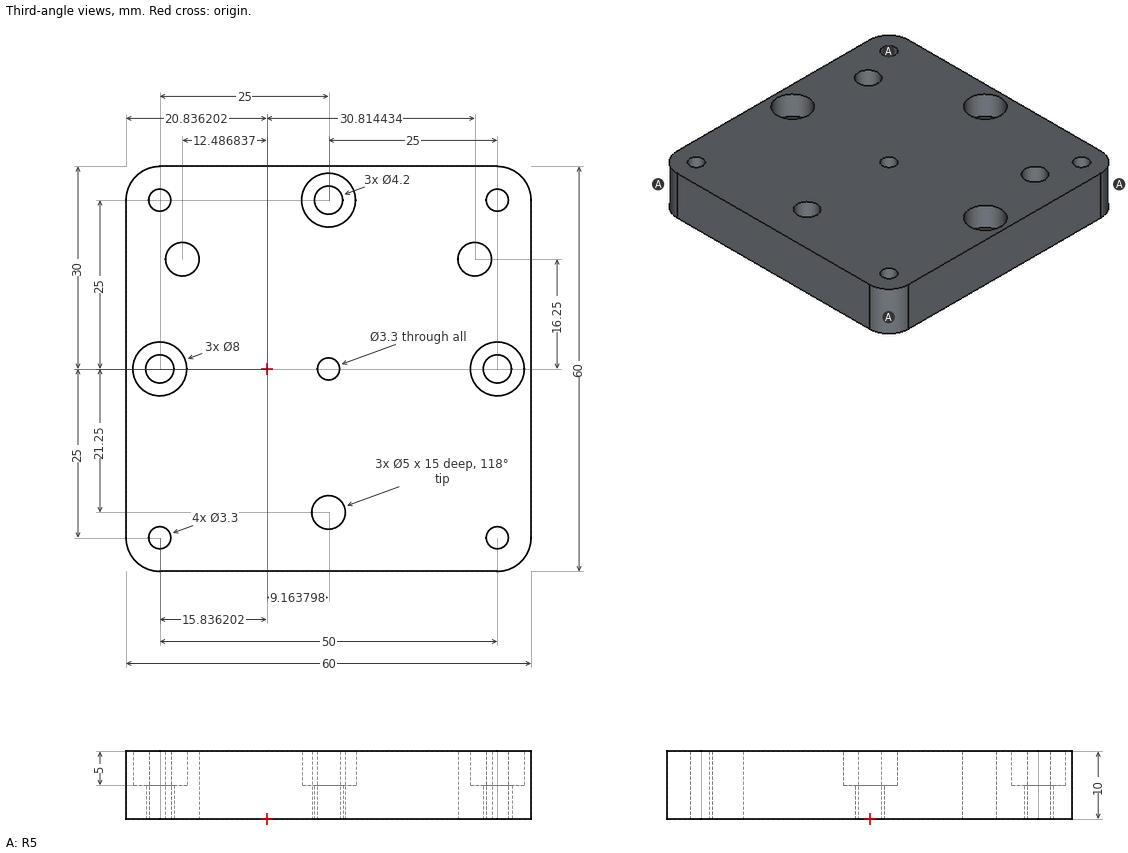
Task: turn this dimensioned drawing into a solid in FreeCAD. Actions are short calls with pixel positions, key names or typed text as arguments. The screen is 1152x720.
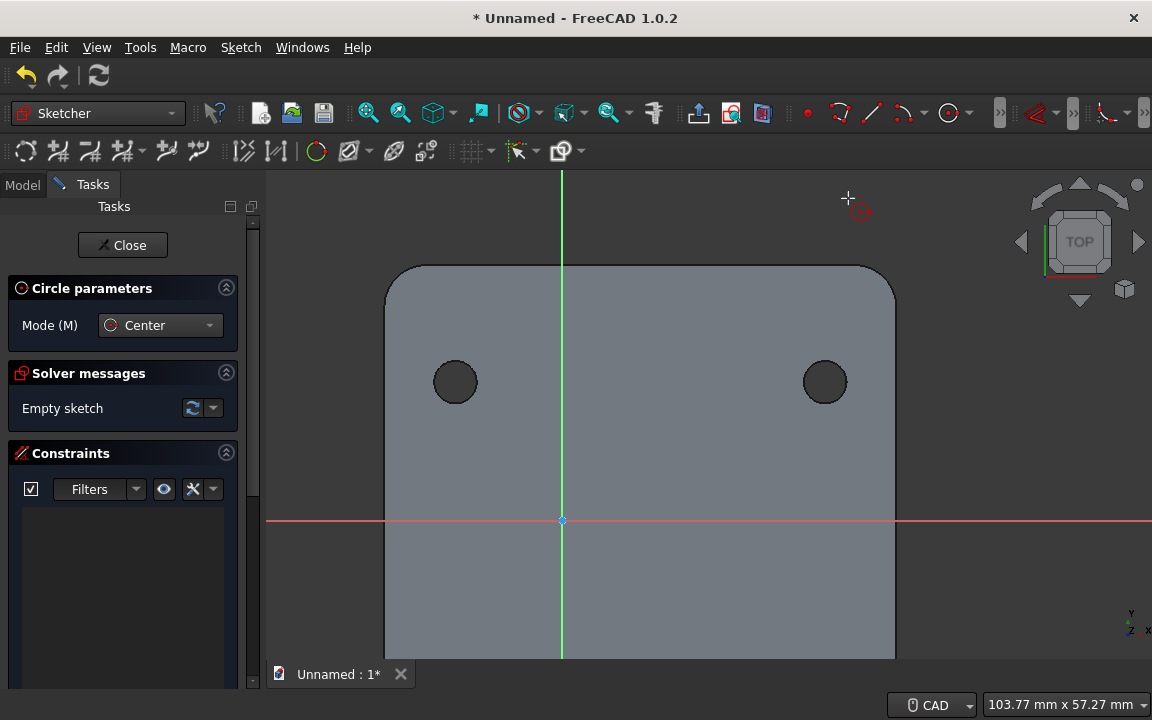
scroll(640, 307, up, 2)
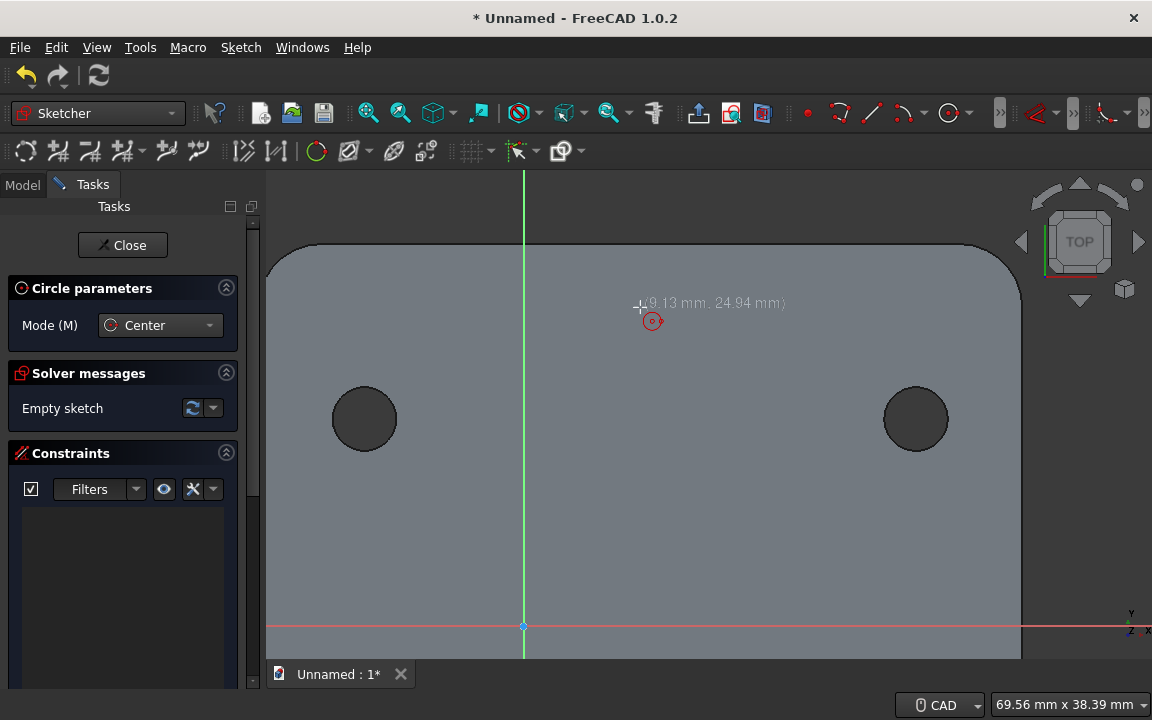
click(640, 308)
move(659, 289)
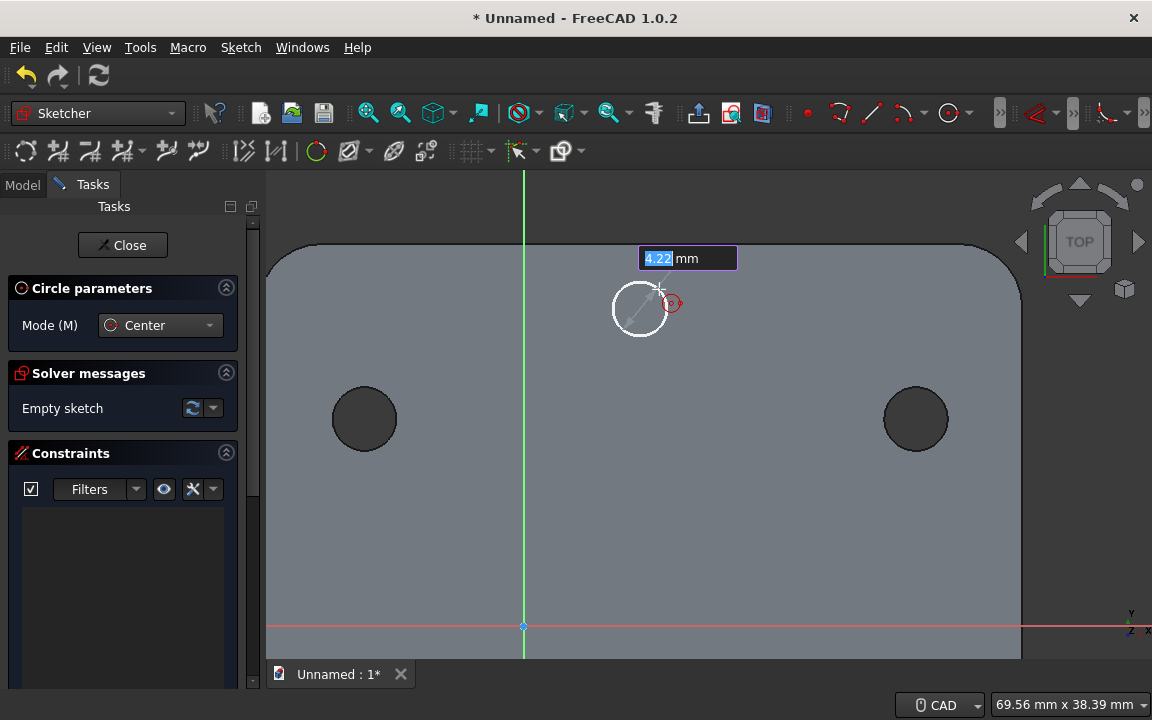
text(4.2)
key(Return)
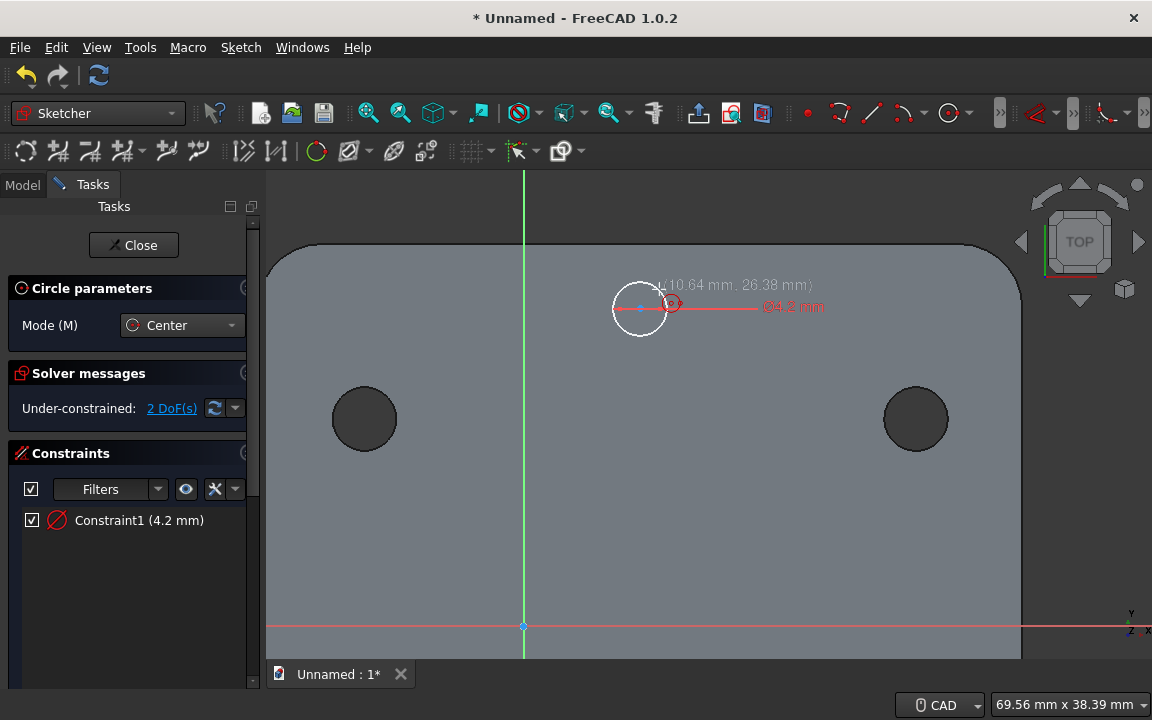
click(959, 626)
move(978, 607)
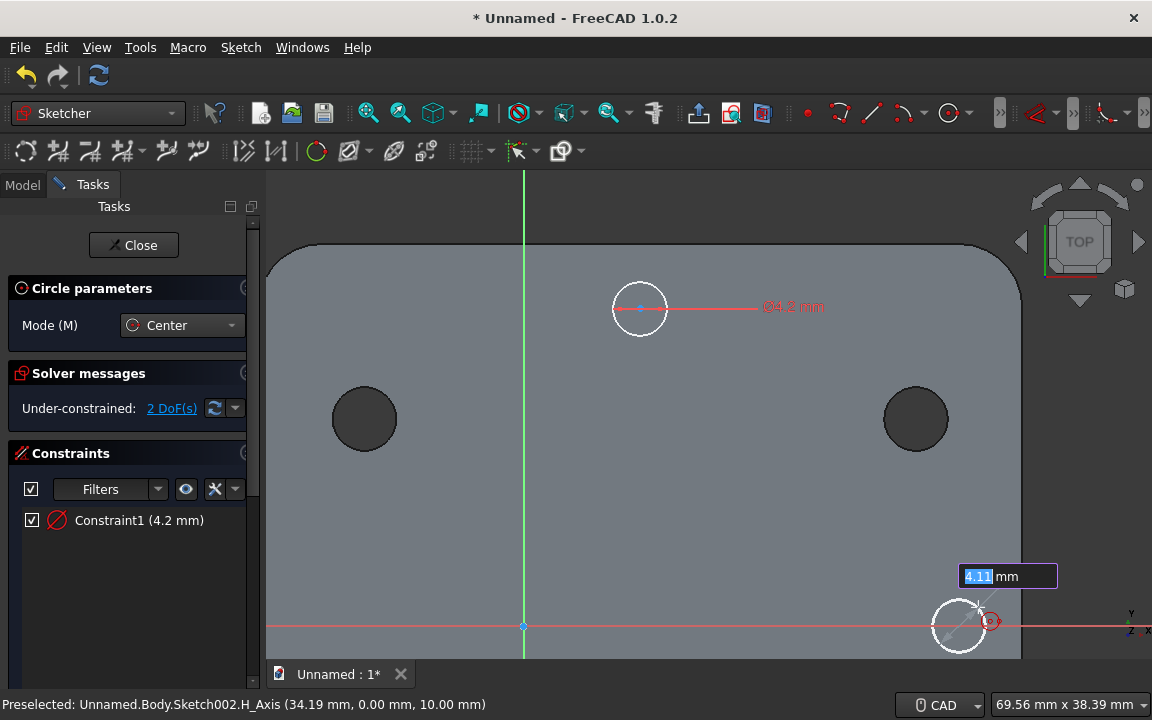
text(4.2)
key(Return)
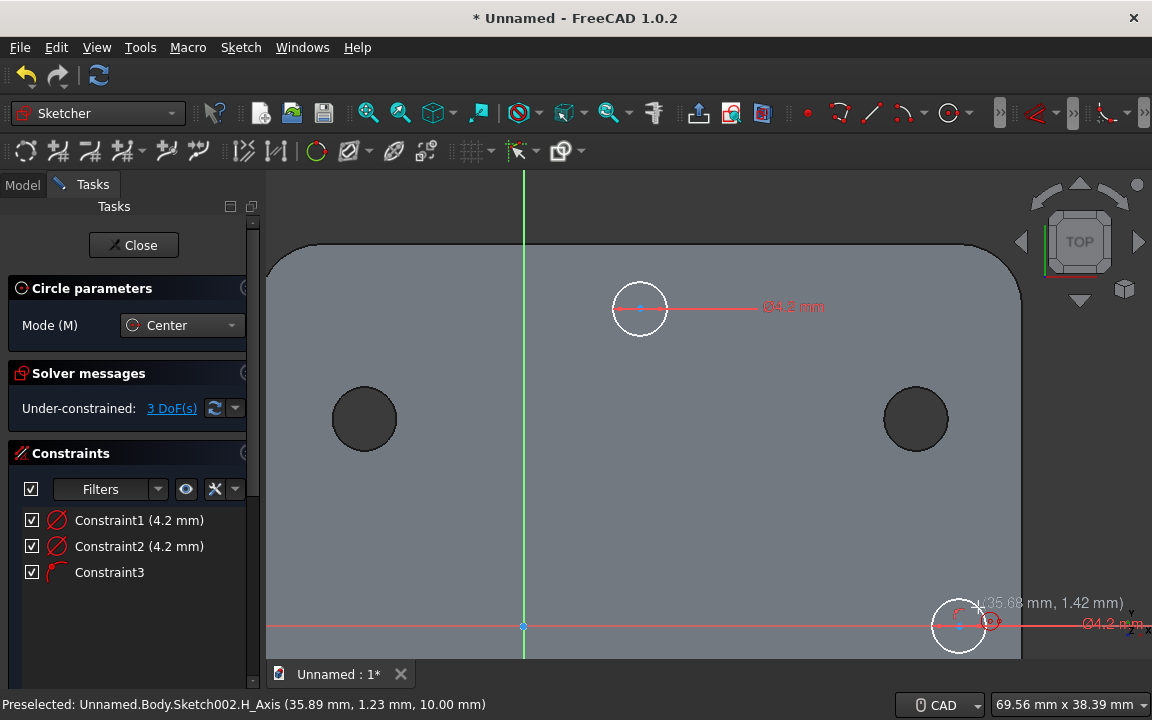
click(322, 626)
move(341, 607)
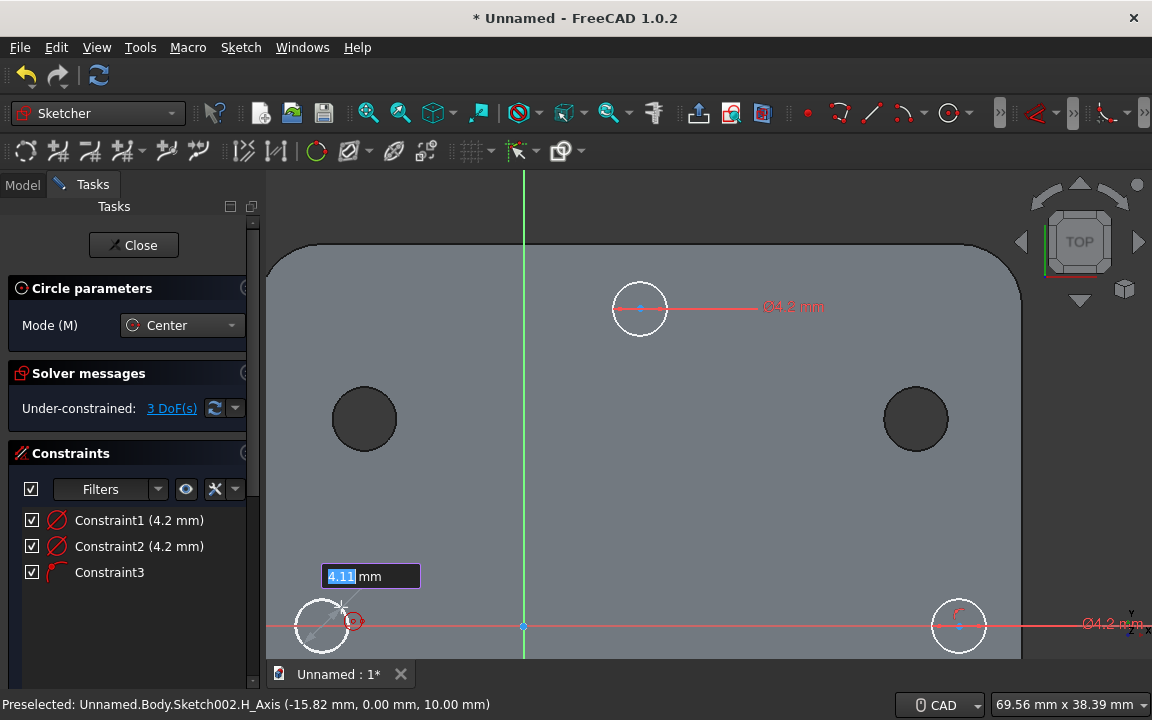
text(4.2)
key(Return)
key(Escape)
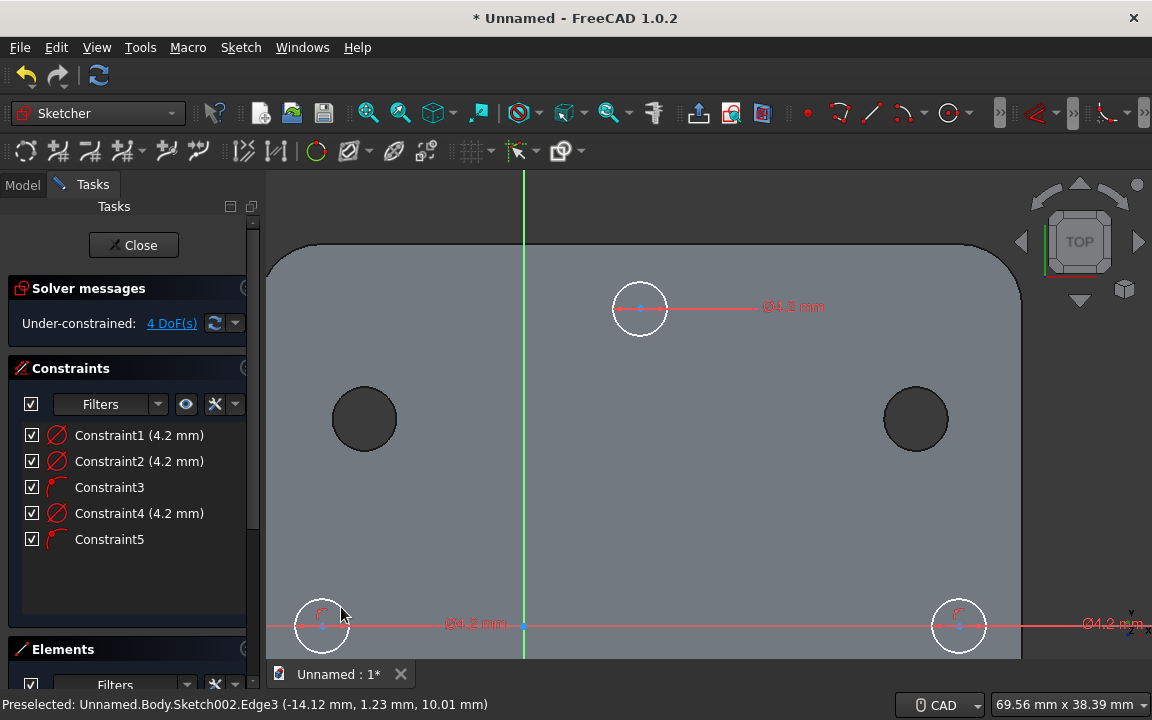
click(1036, 114)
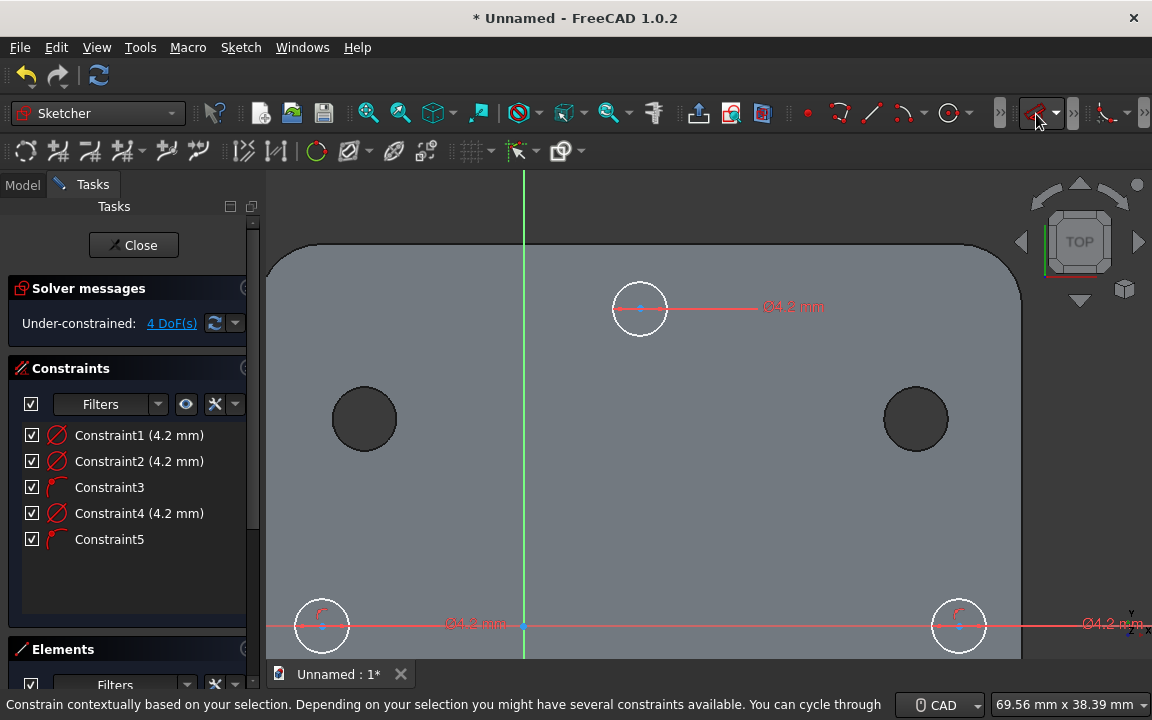
click(640, 309)
click(490, 468)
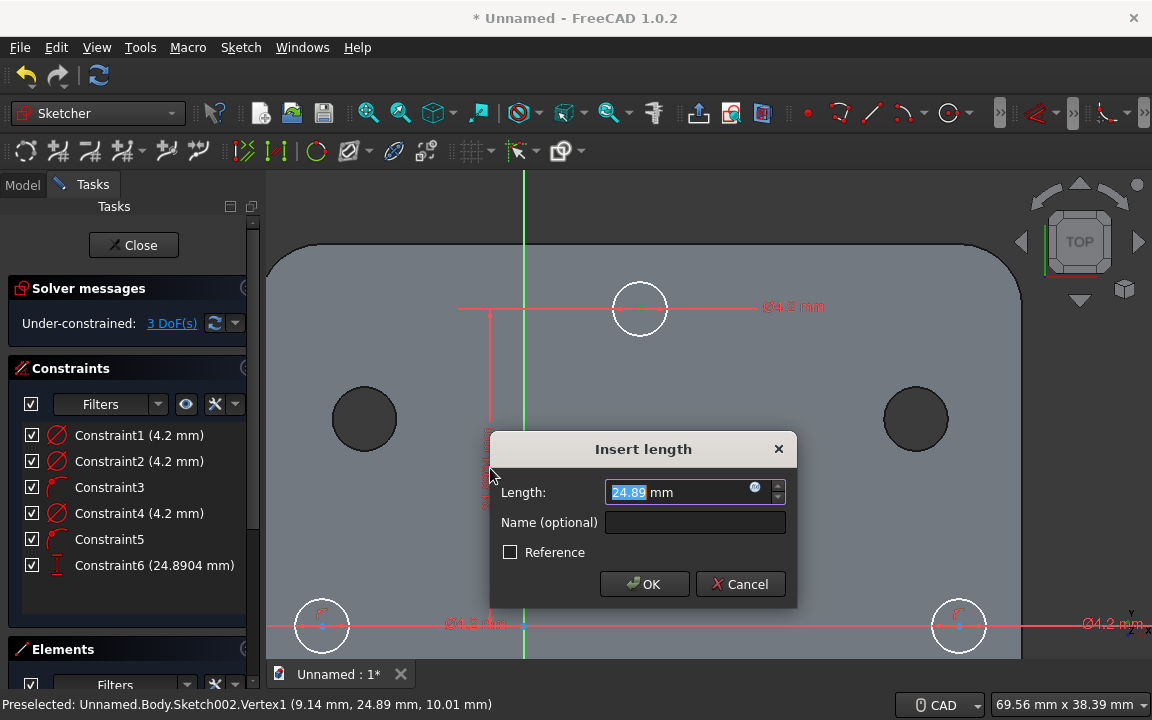
text(25)
key(Return)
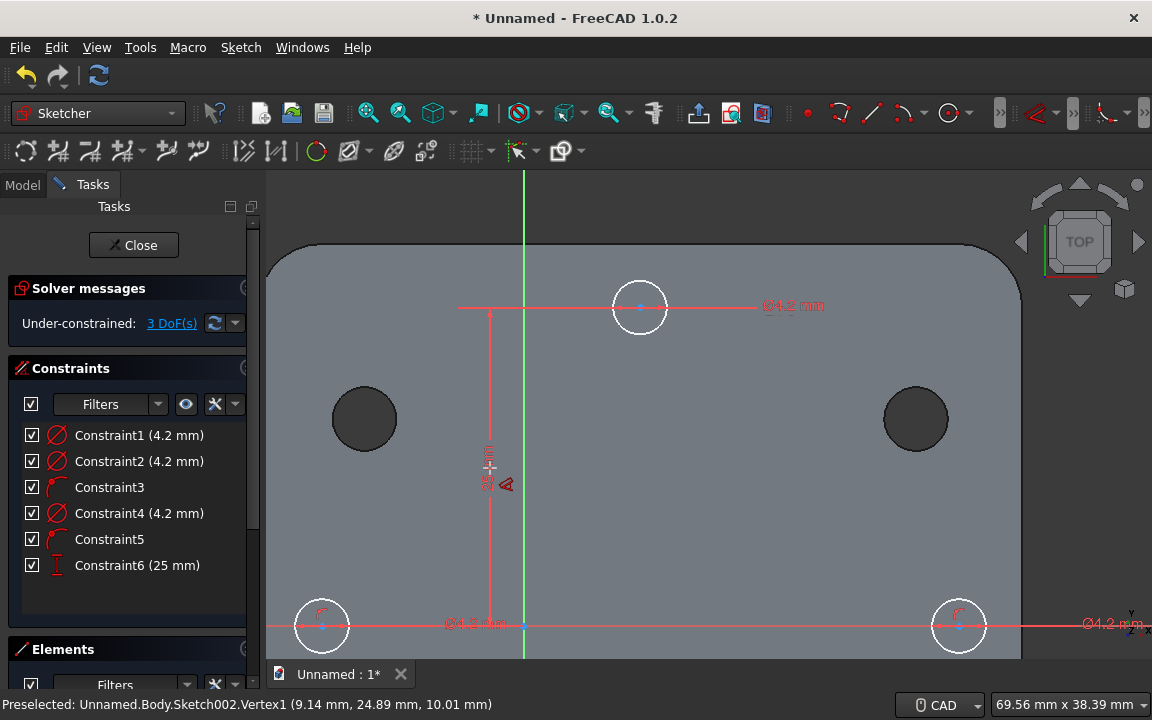
click(640, 308)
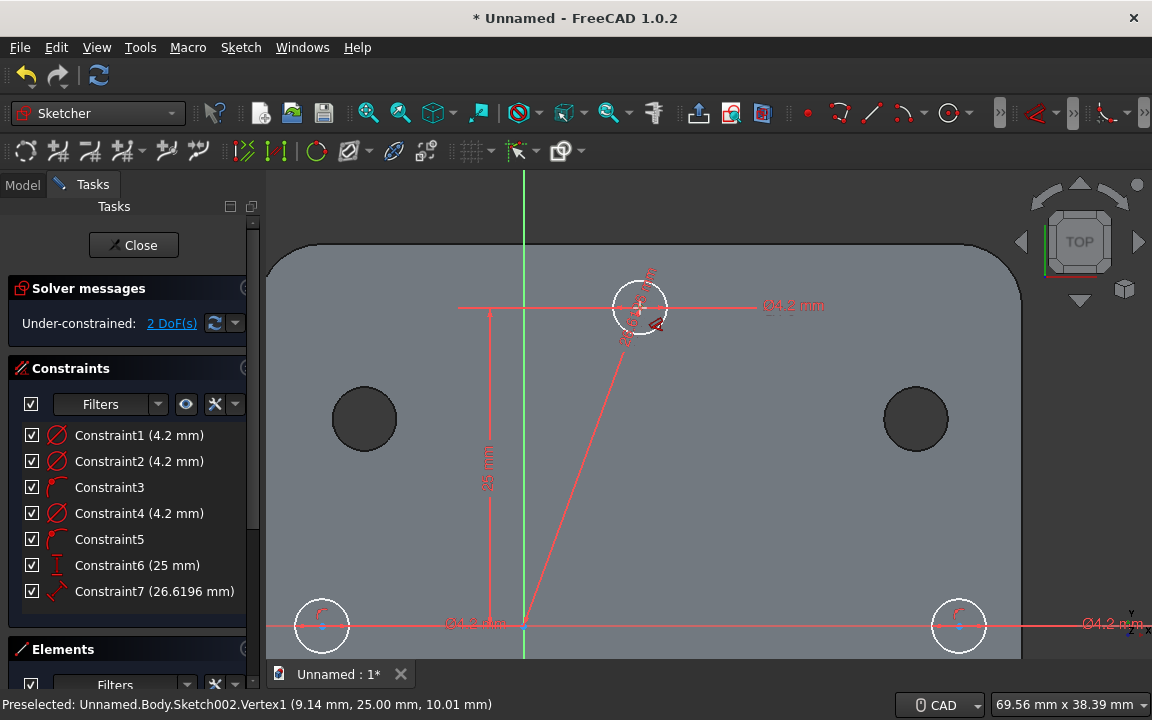
click(959, 626)
click(799, 274)